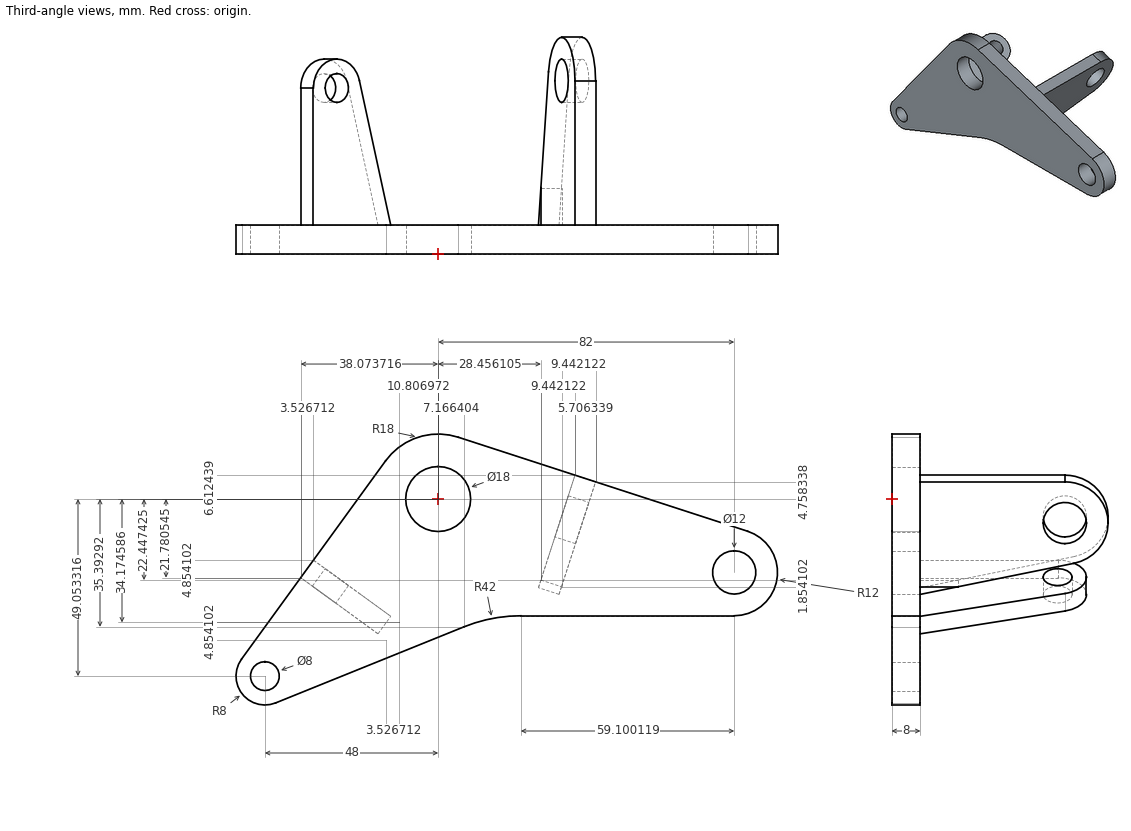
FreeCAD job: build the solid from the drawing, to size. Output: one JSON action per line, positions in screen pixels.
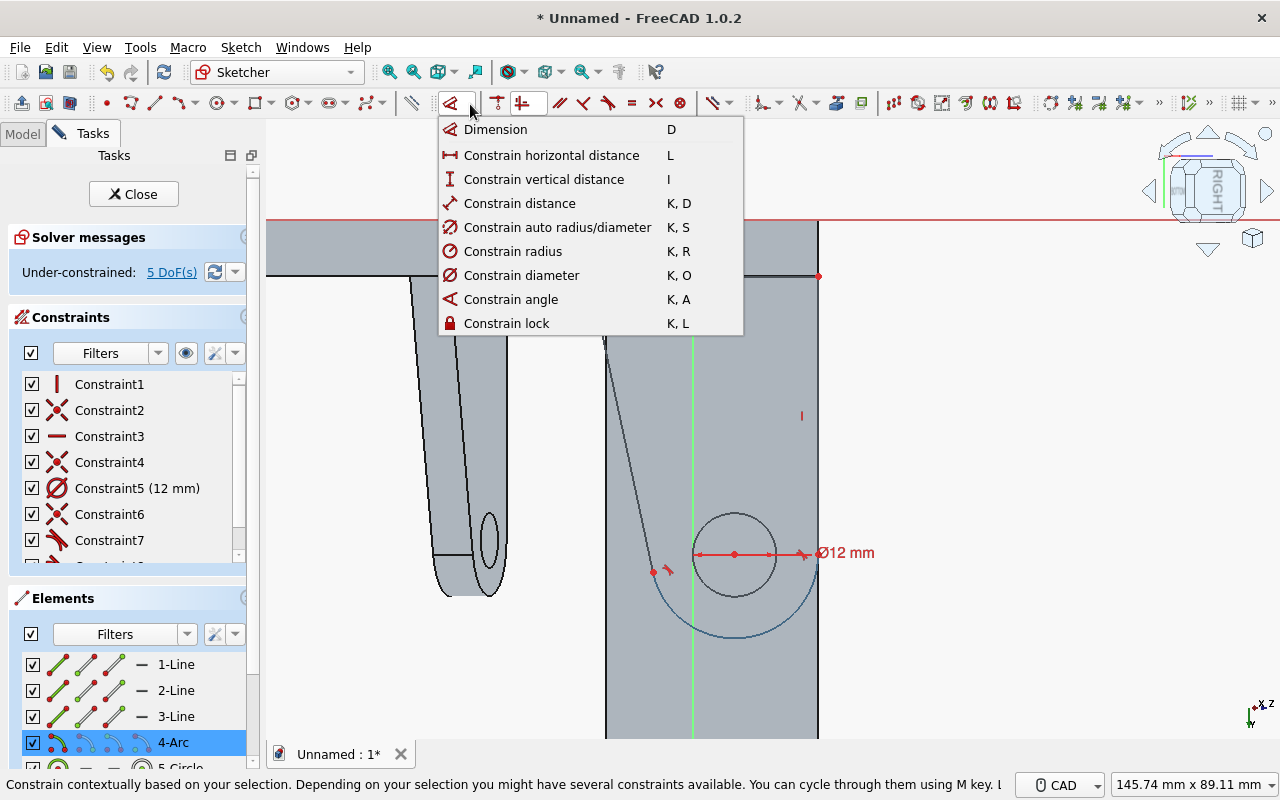
{"action": "left_click", "coordinate": [591, 251]}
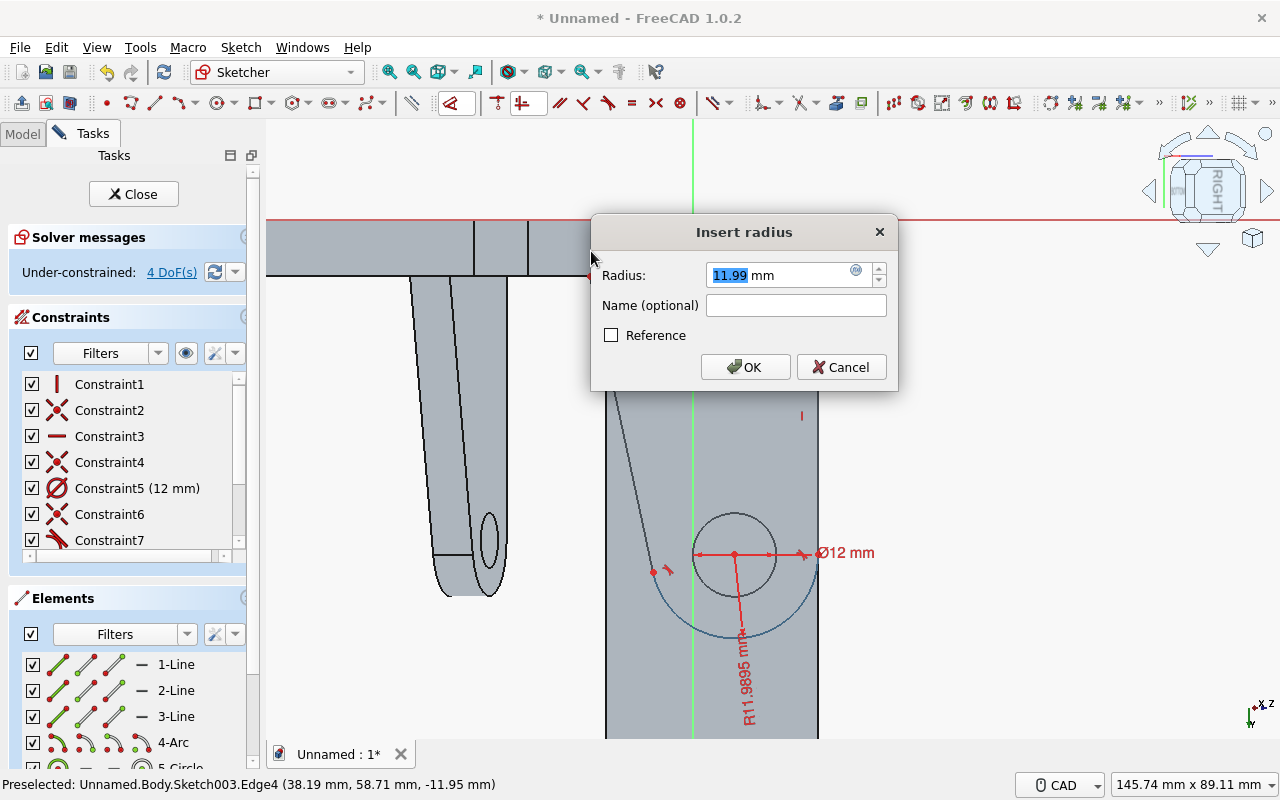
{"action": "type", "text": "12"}
{"action": "key", "text": "Return"}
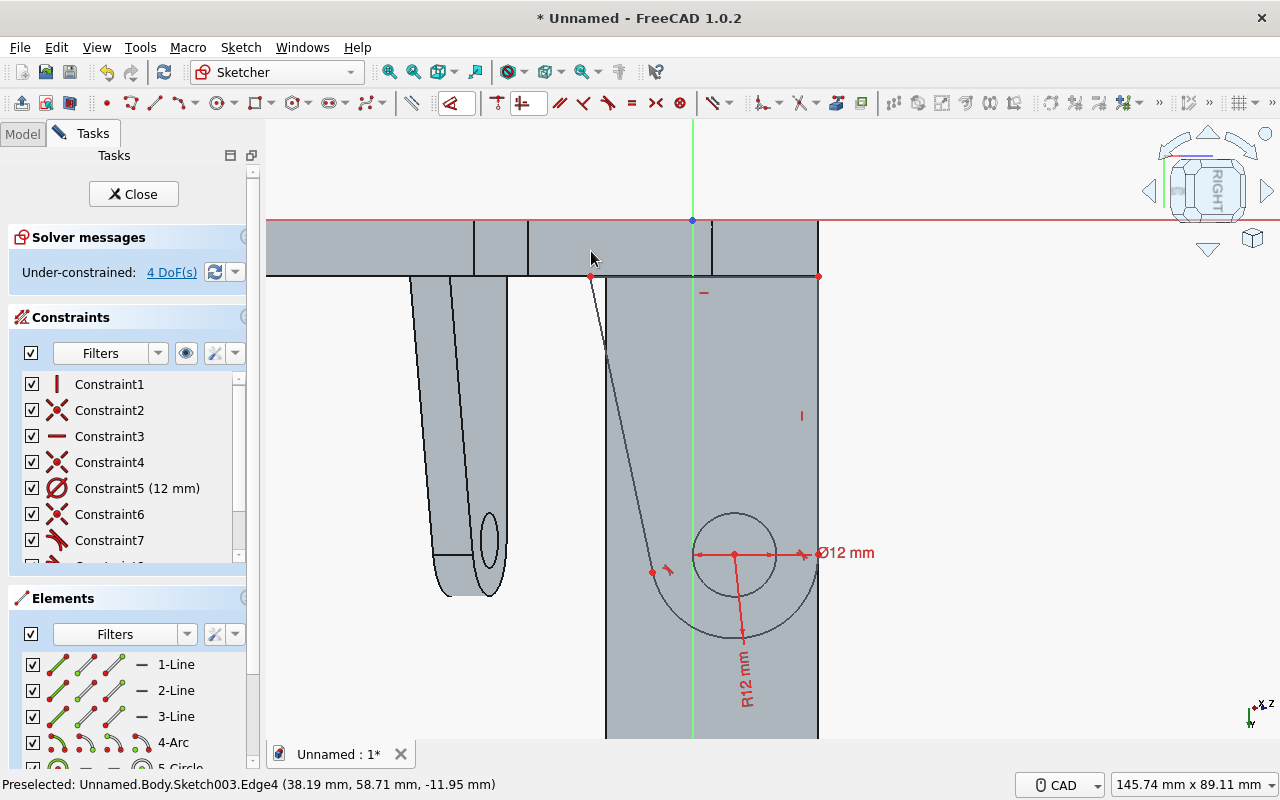
{"action": "left_click", "coordinate": [818, 472]}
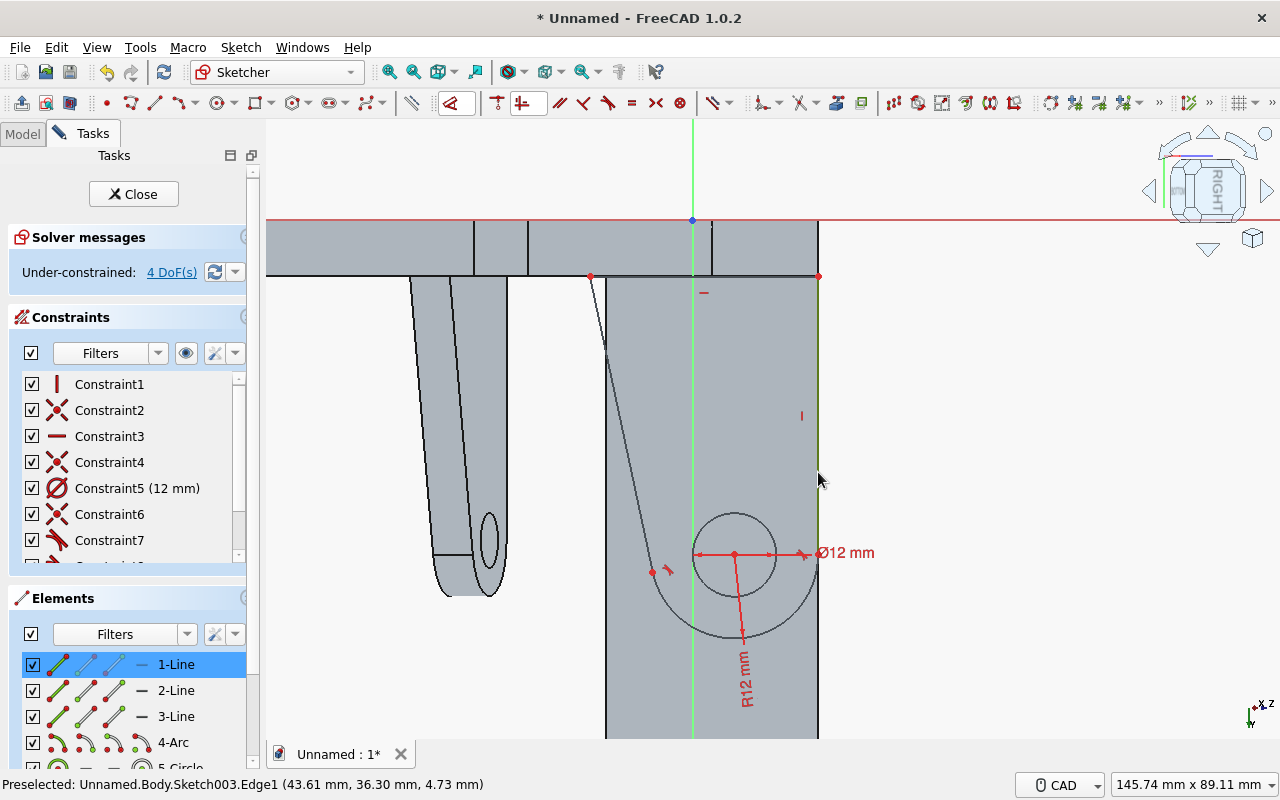
{"action": "left_click", "coordinate": [470, 104]}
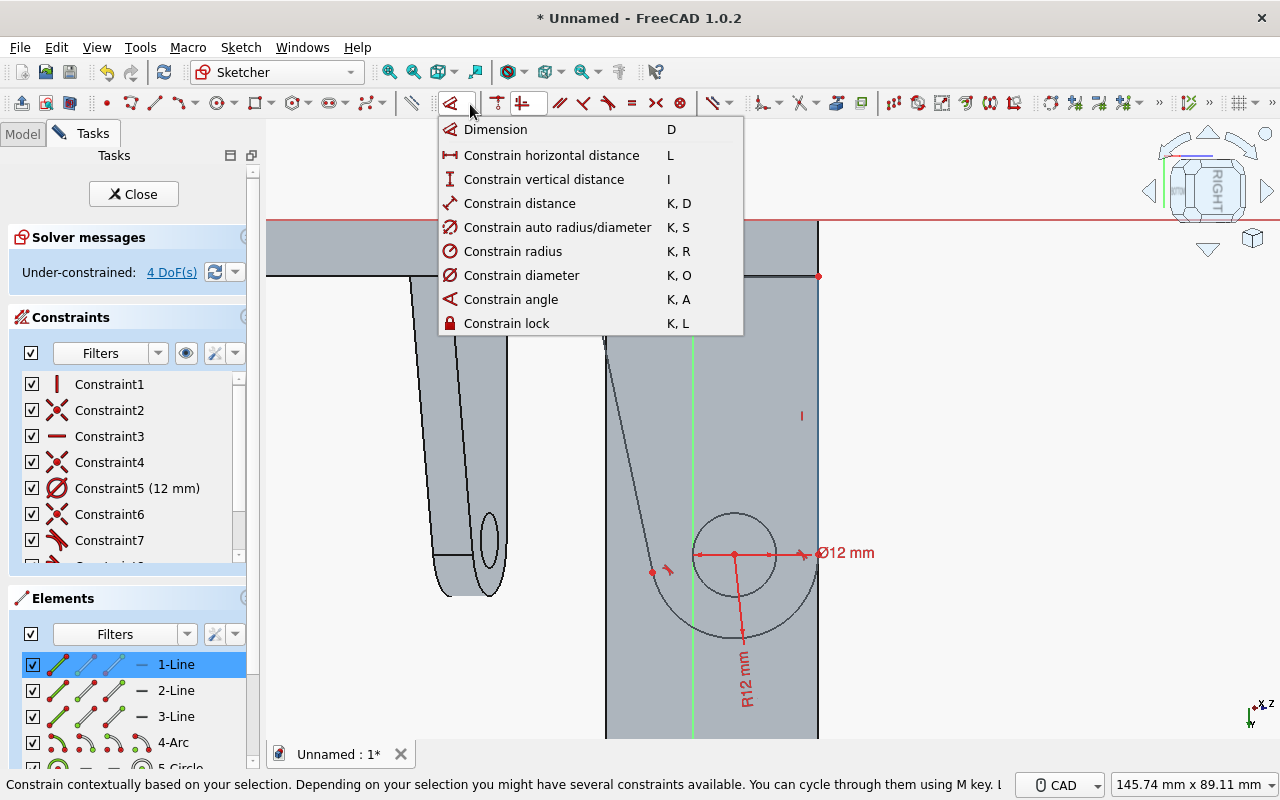
{"action": "left_click", "coordinate": [591, 179]}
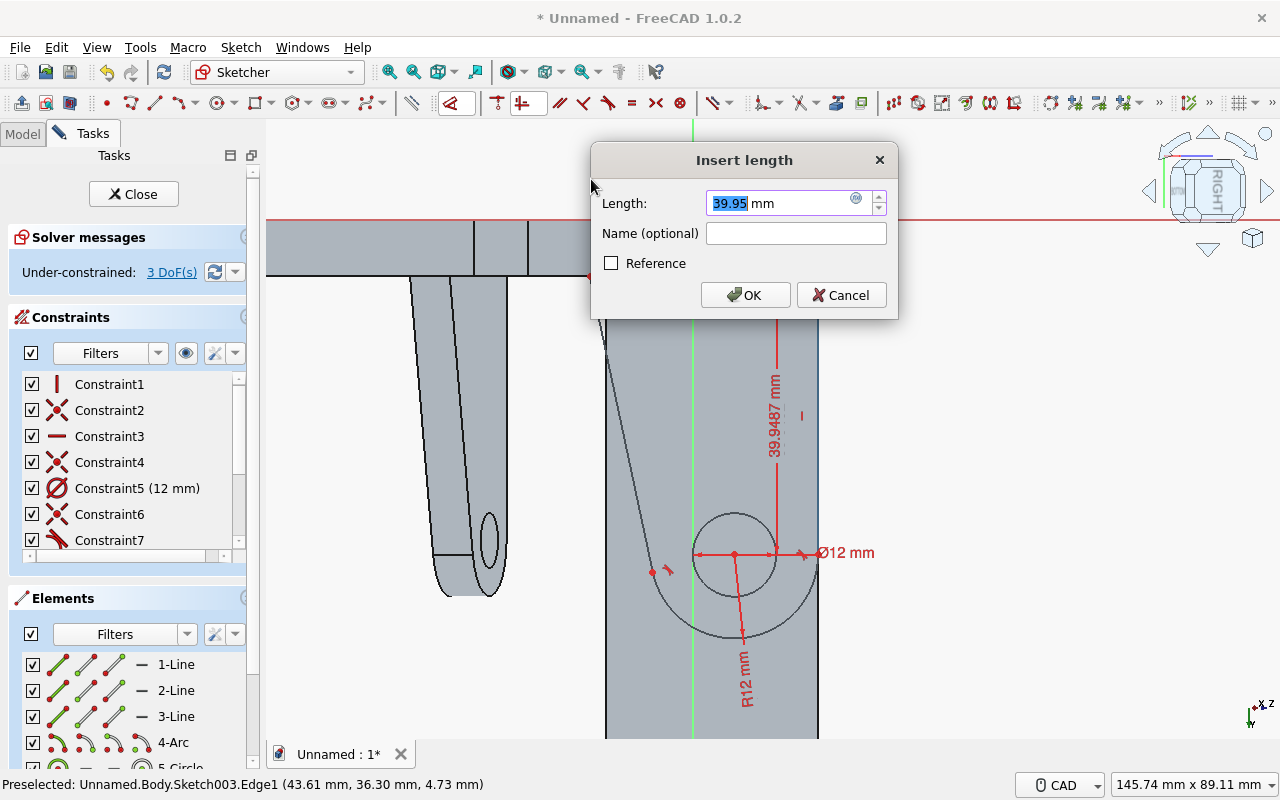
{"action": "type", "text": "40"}
{"action": "key", "text": "Return"}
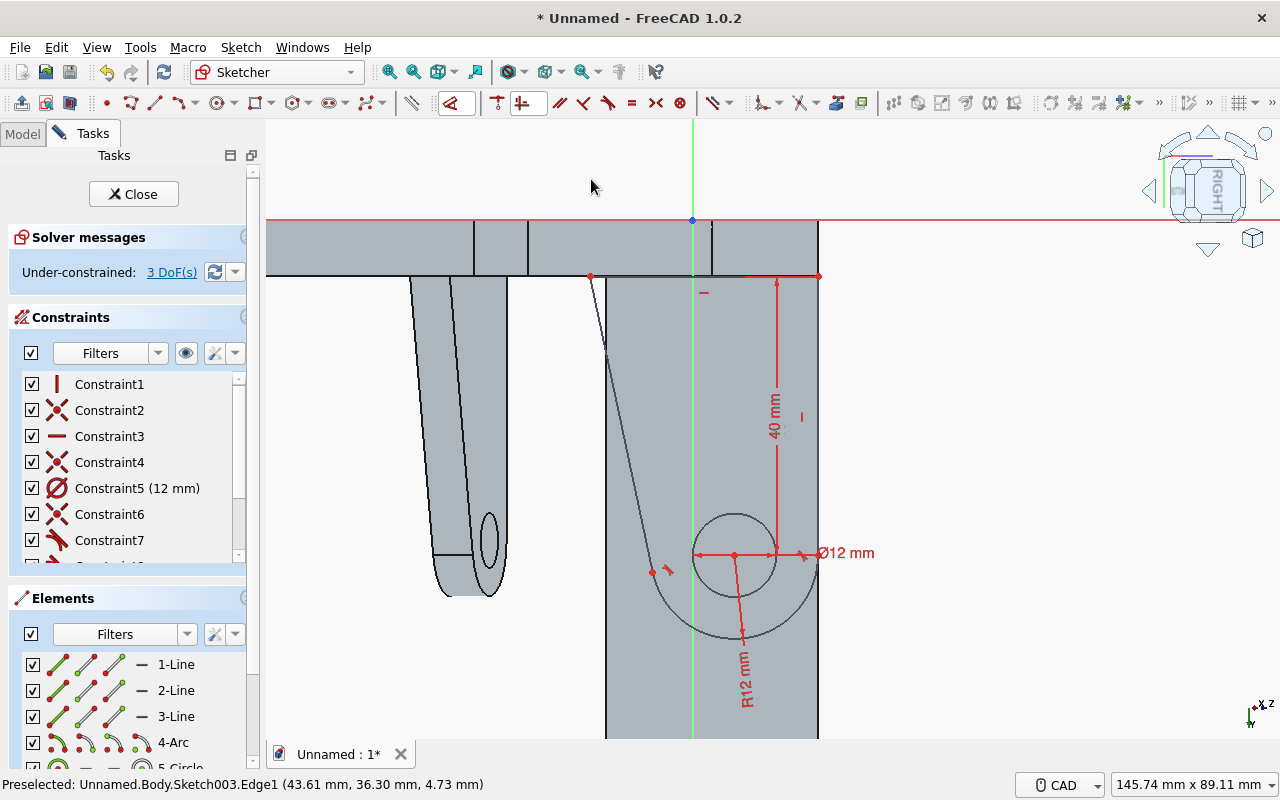
{"action": "left_click", "coordinate": [818, 277]}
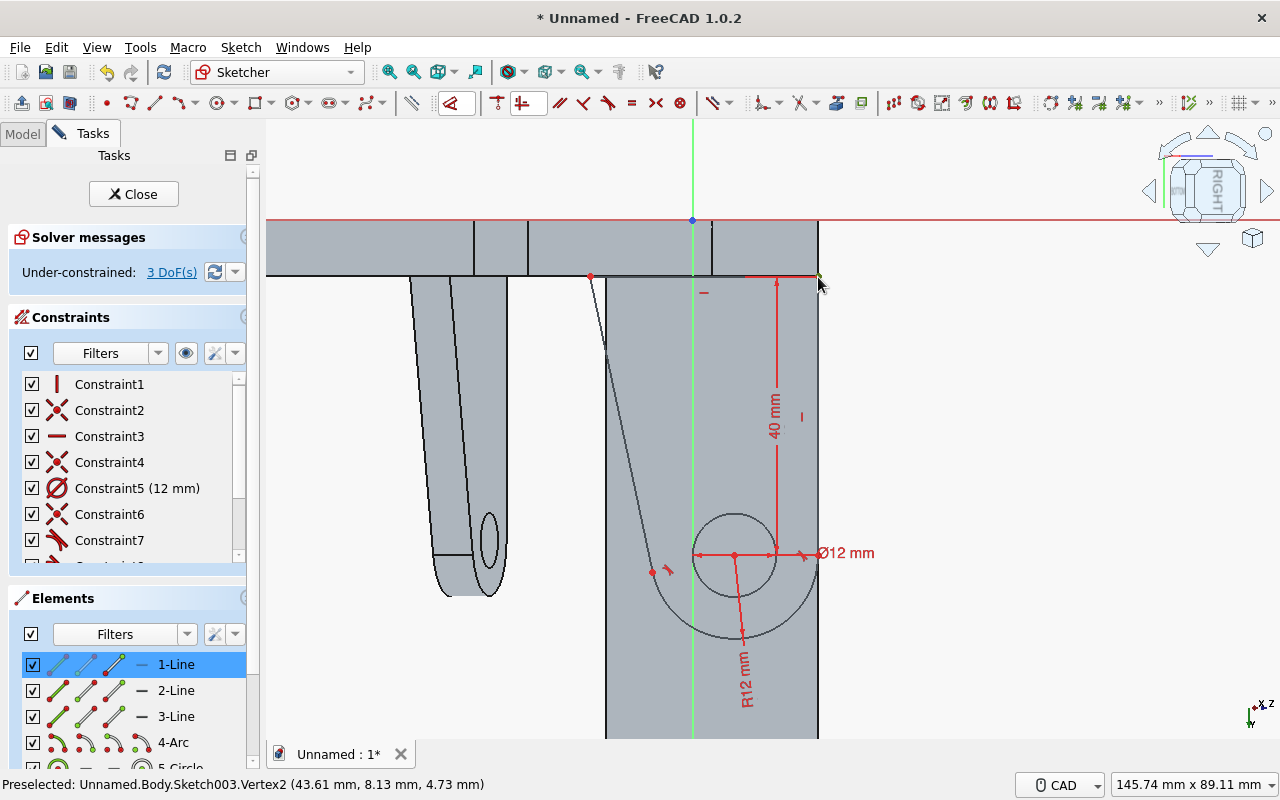
{"action": "left_click", "coordinate": [470, 104]}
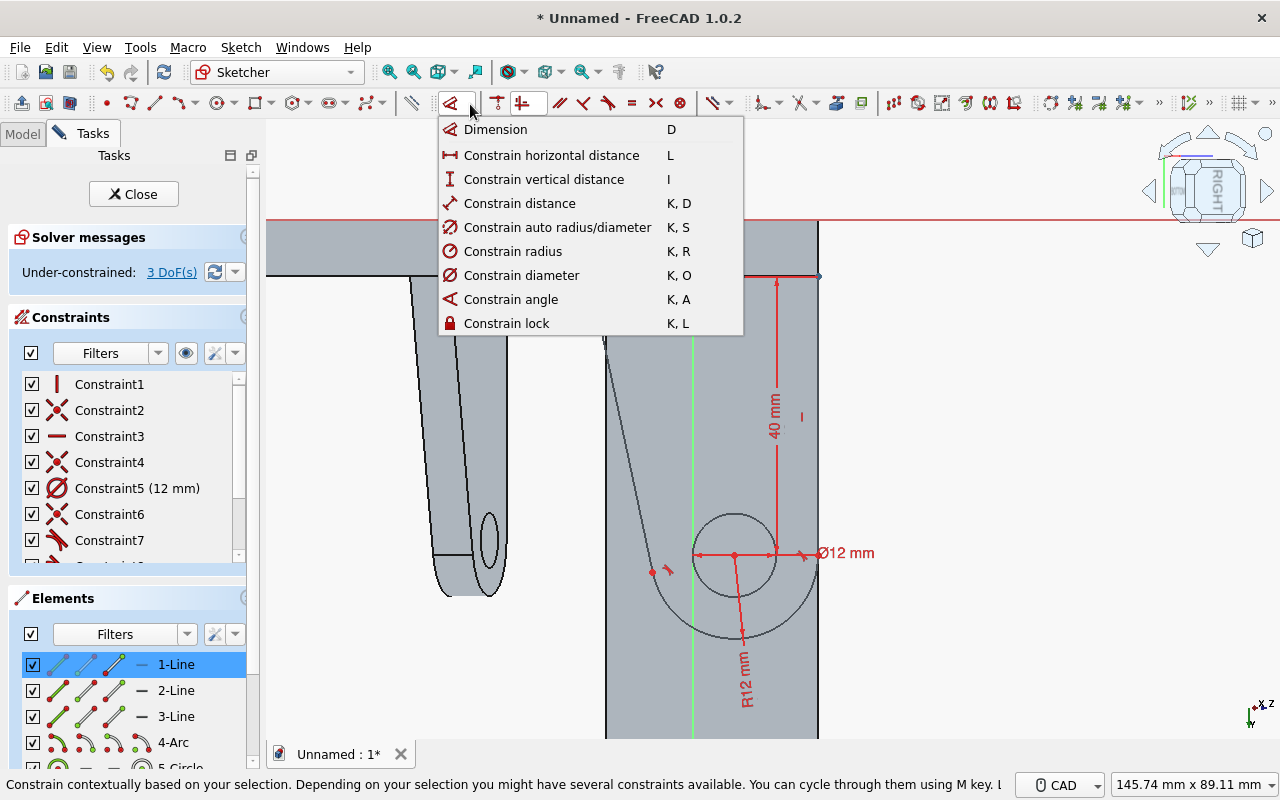
{"action": "left_click", "coordinate": [591, 179]}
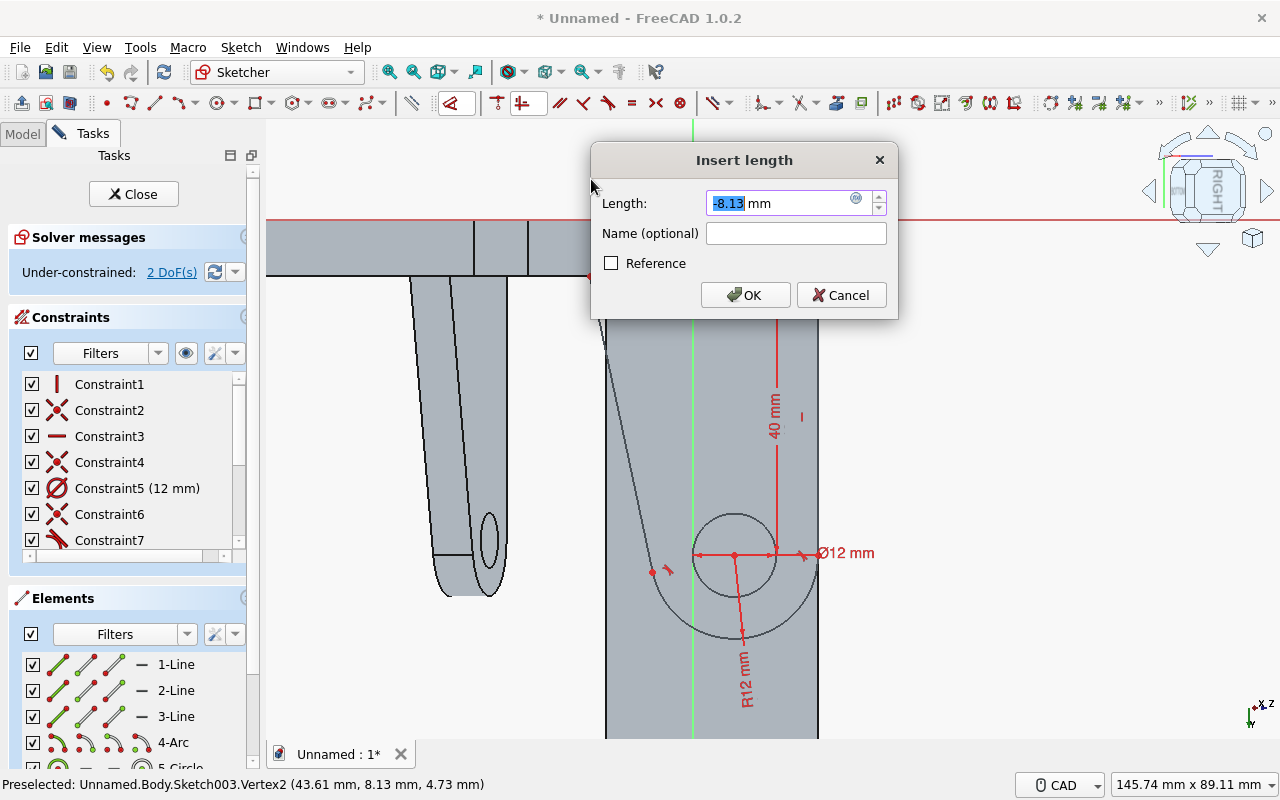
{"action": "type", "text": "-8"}
{"action": "key", "text": "Return"}